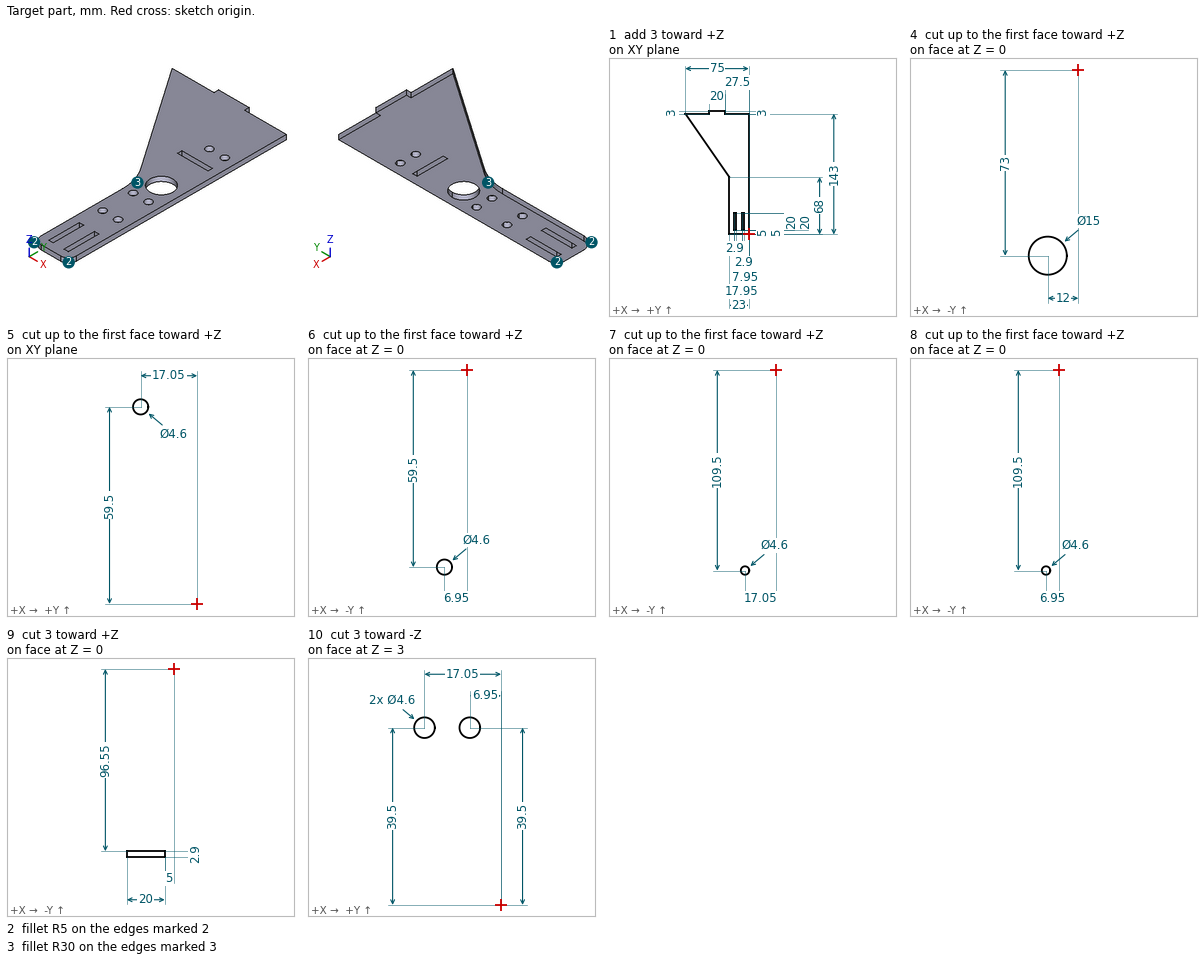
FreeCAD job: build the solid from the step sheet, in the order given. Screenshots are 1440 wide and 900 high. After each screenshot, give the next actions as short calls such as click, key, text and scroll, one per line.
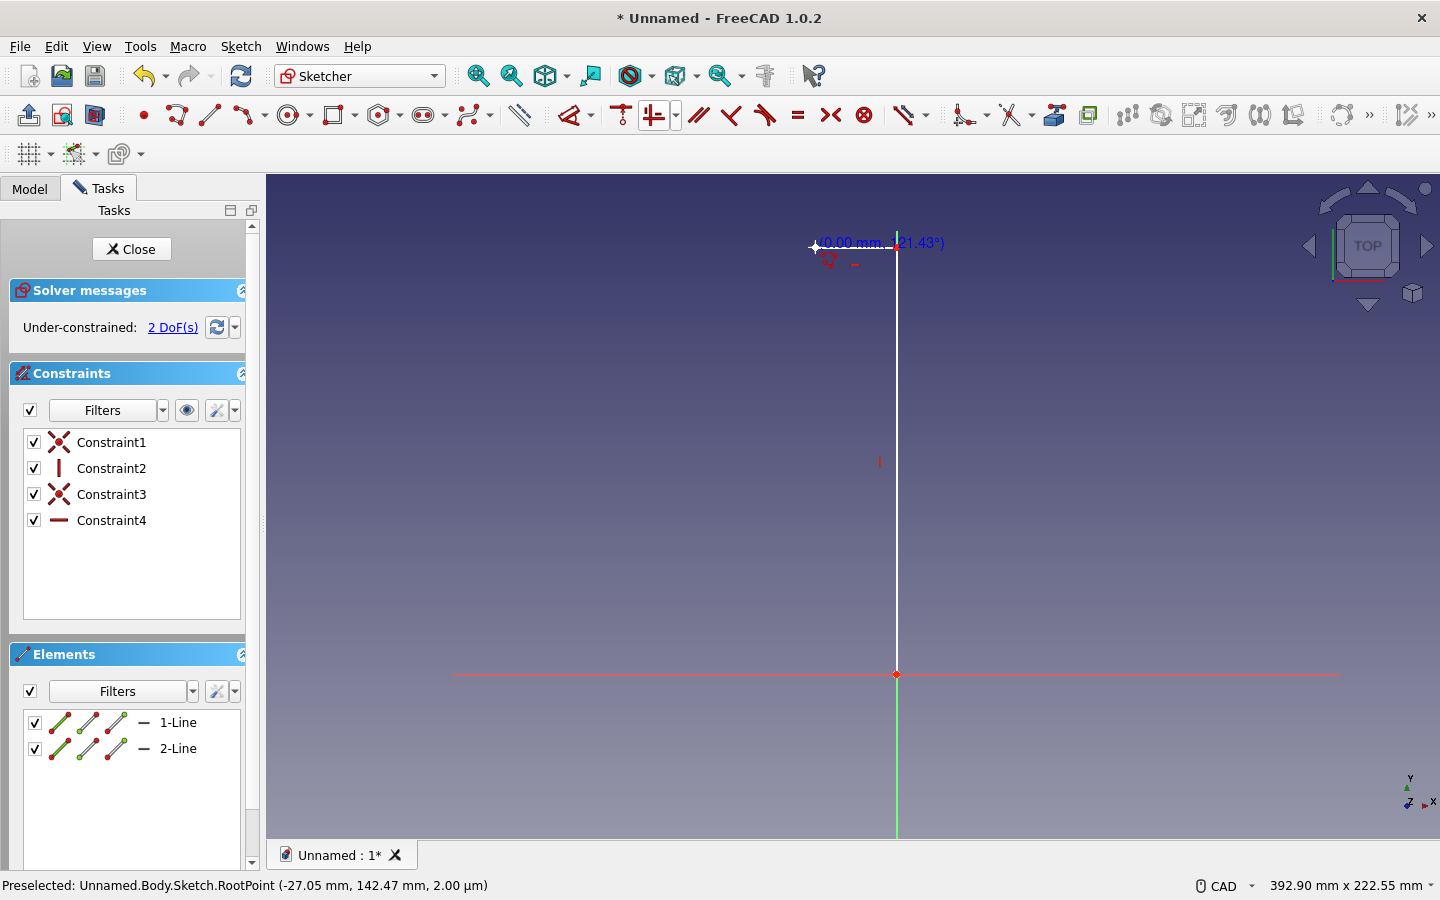
scroll(815, 238, up, 3)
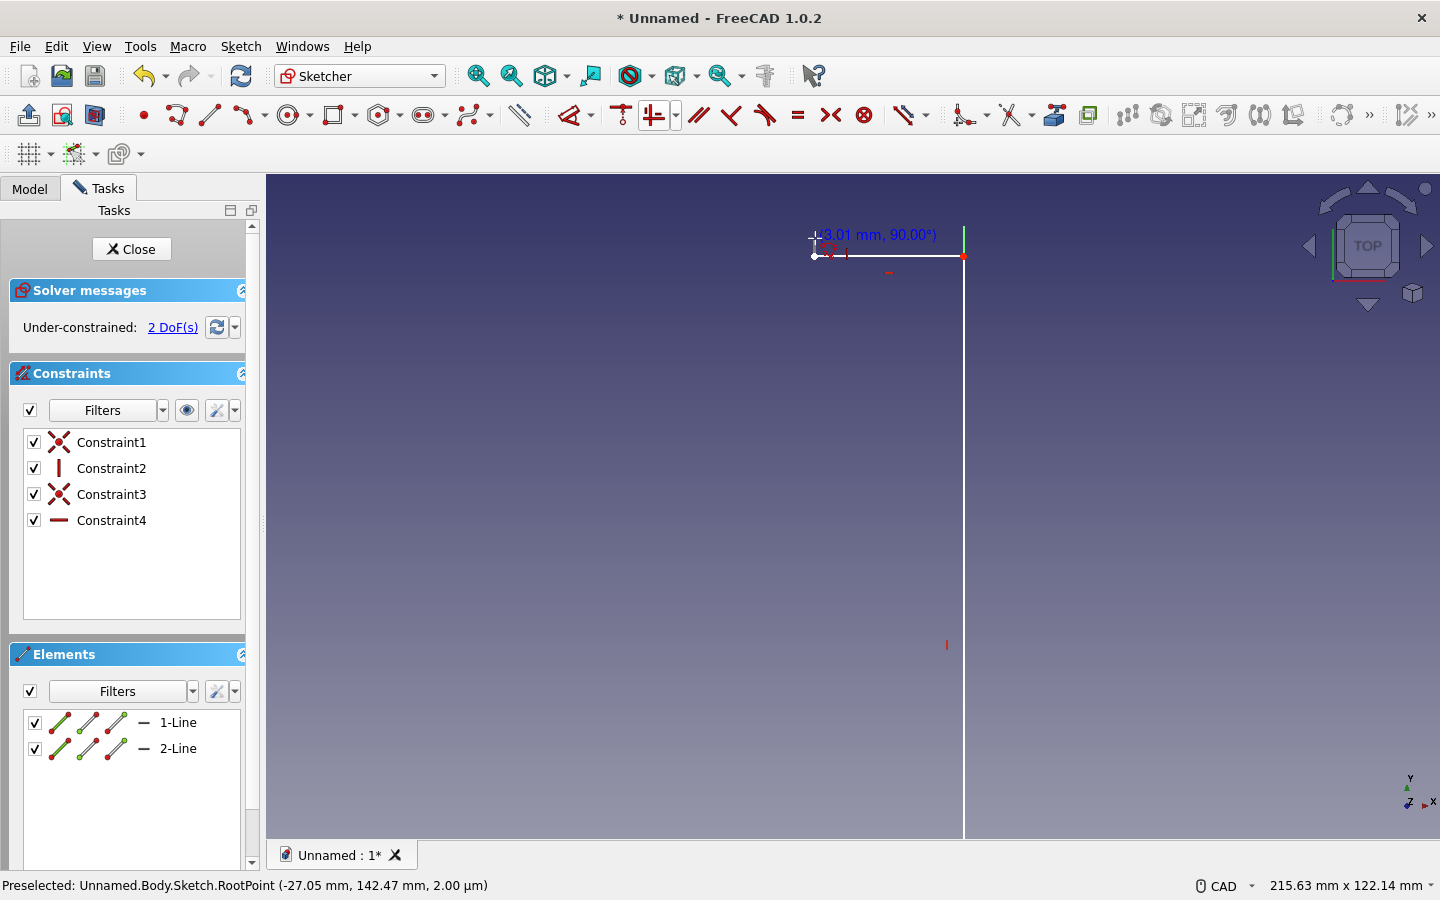
click(815, 239)
click(705, 239)
click(705, 255)
click(555, 255)
click(838, 663)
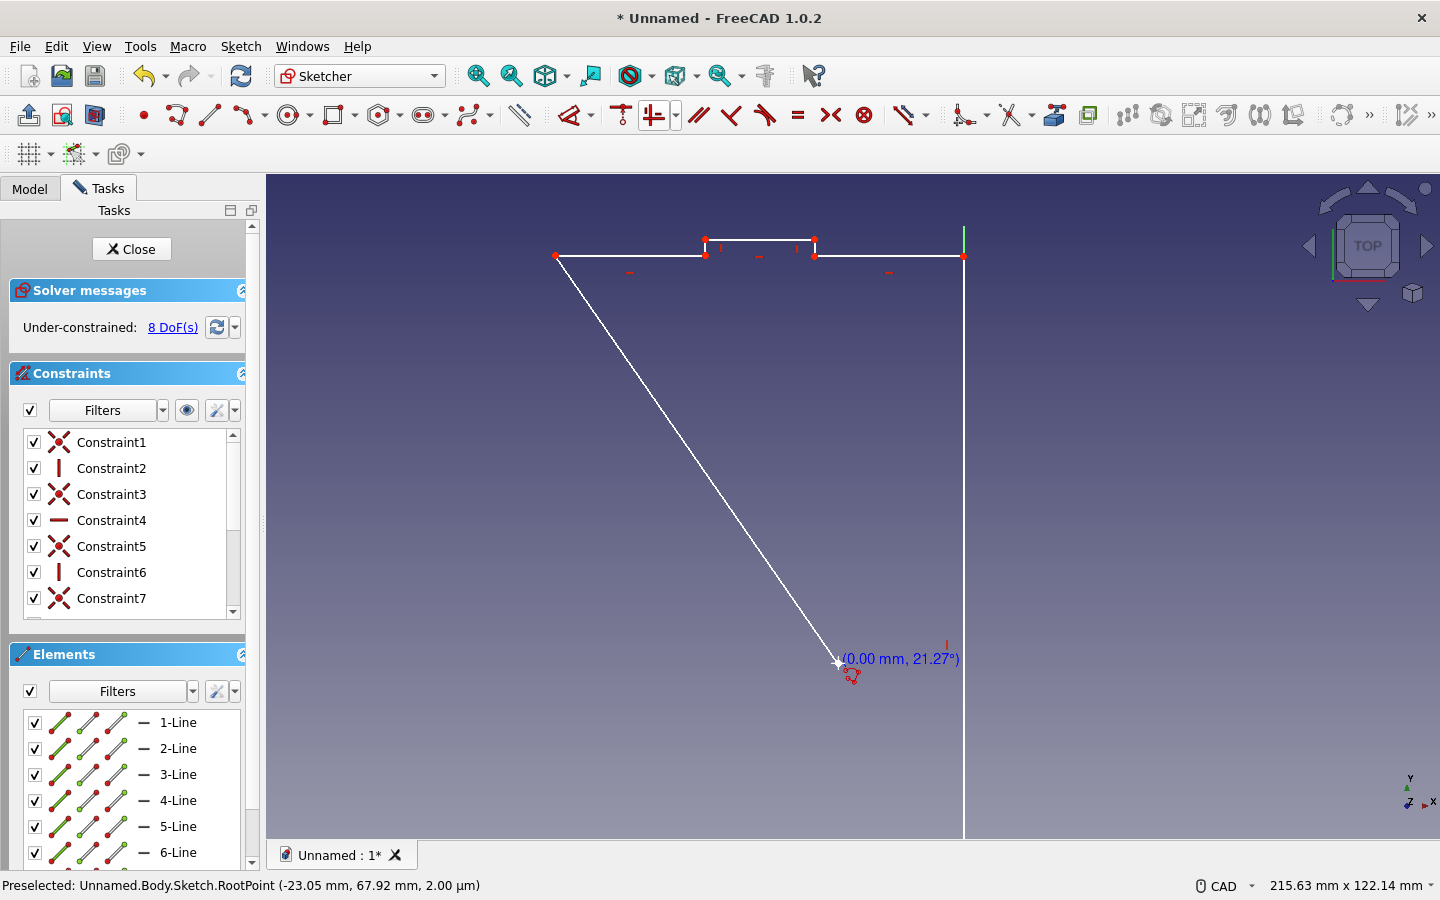
scroll(815, 349, down, 3)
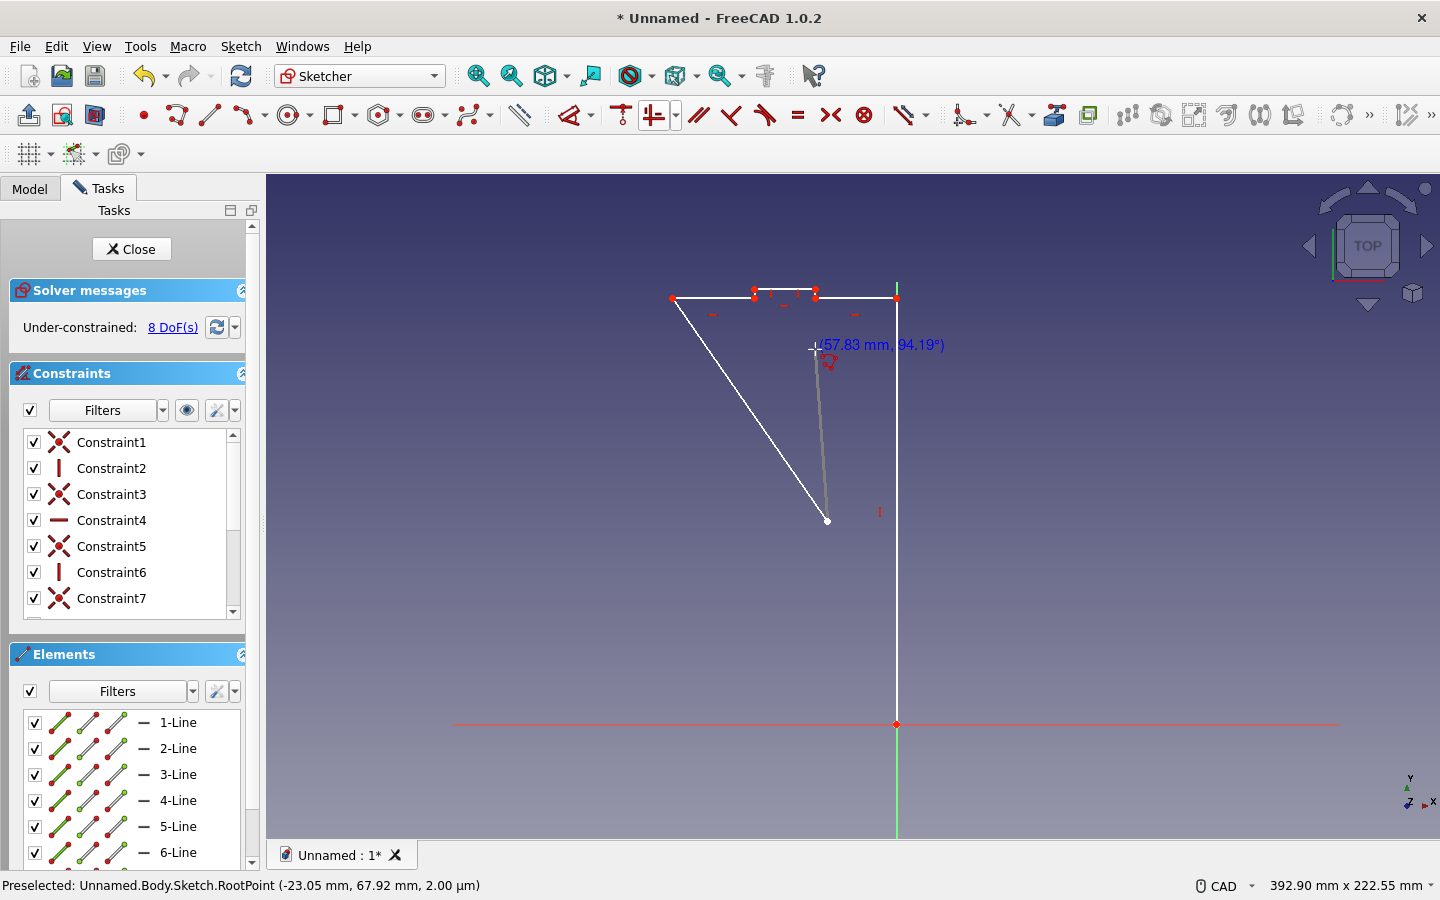
click(828, 716)
click(897, 725)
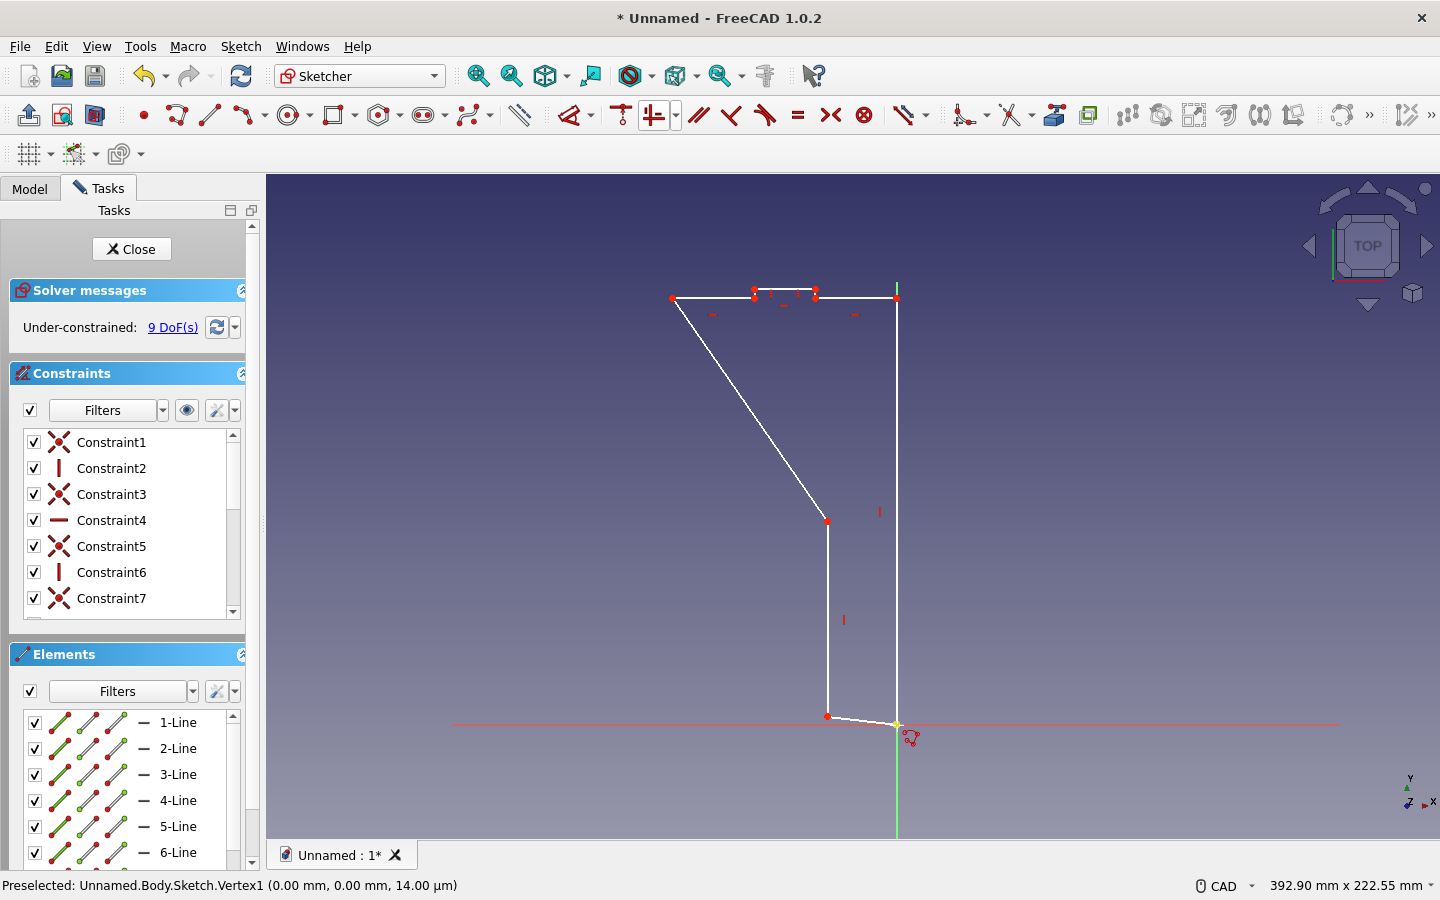
key(g)
key(r)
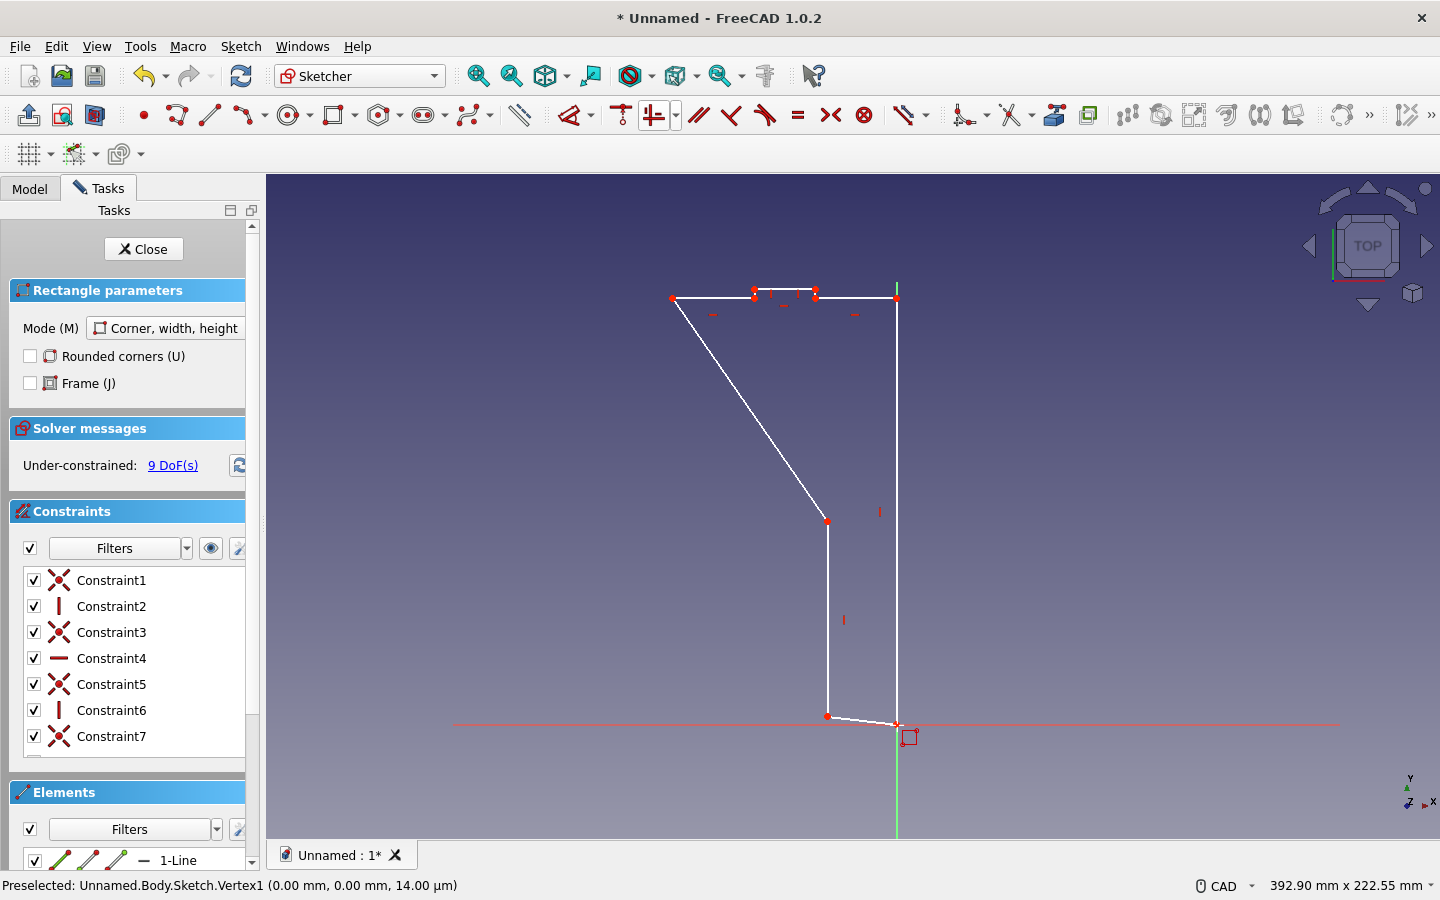
scroll(873, 650, up, 4)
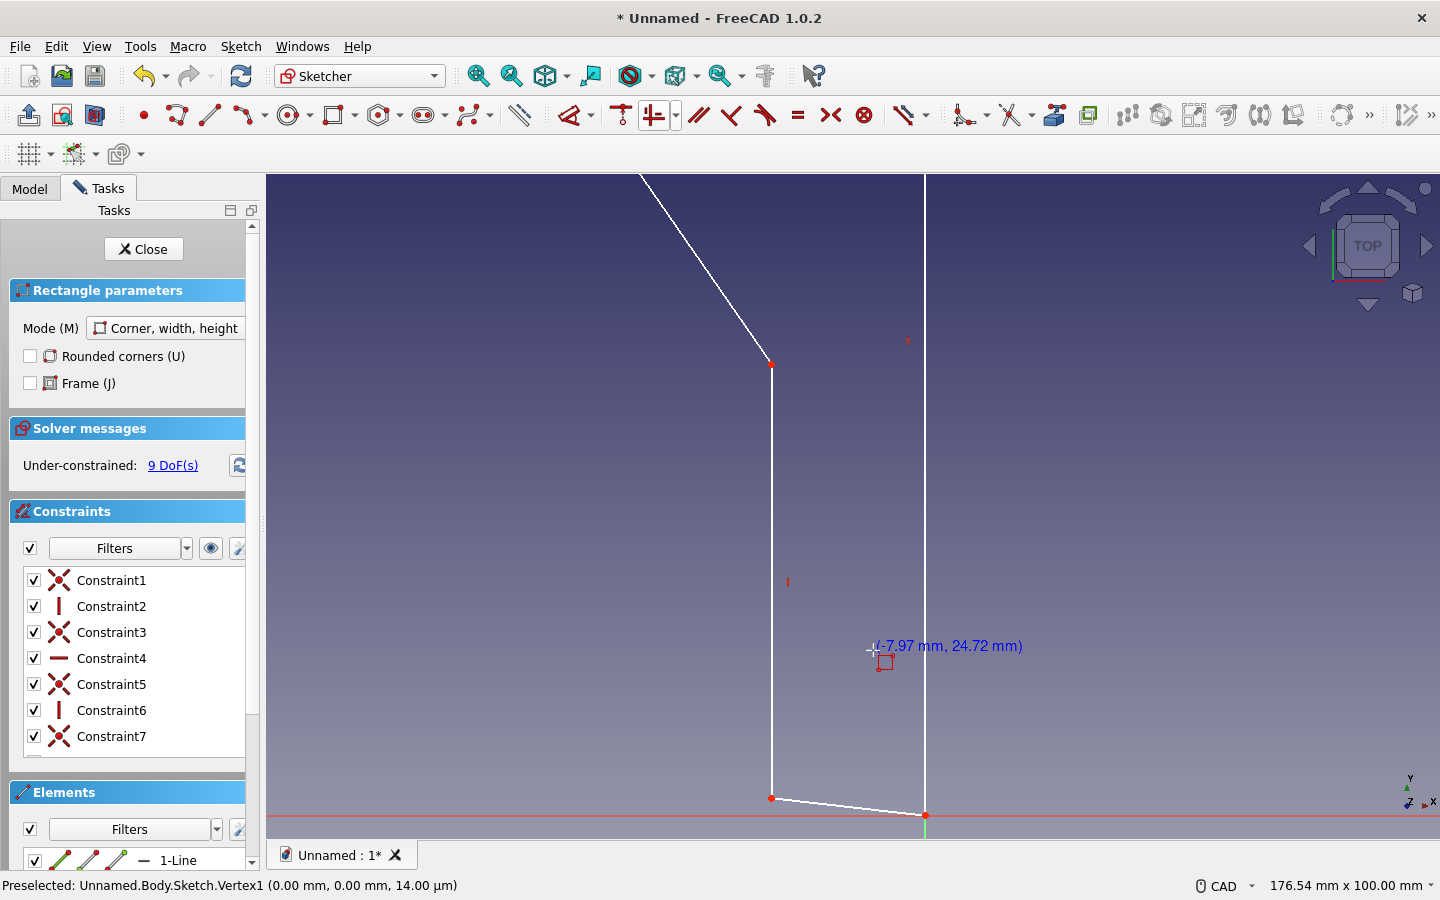
click(873, 649)
move(892, 782)